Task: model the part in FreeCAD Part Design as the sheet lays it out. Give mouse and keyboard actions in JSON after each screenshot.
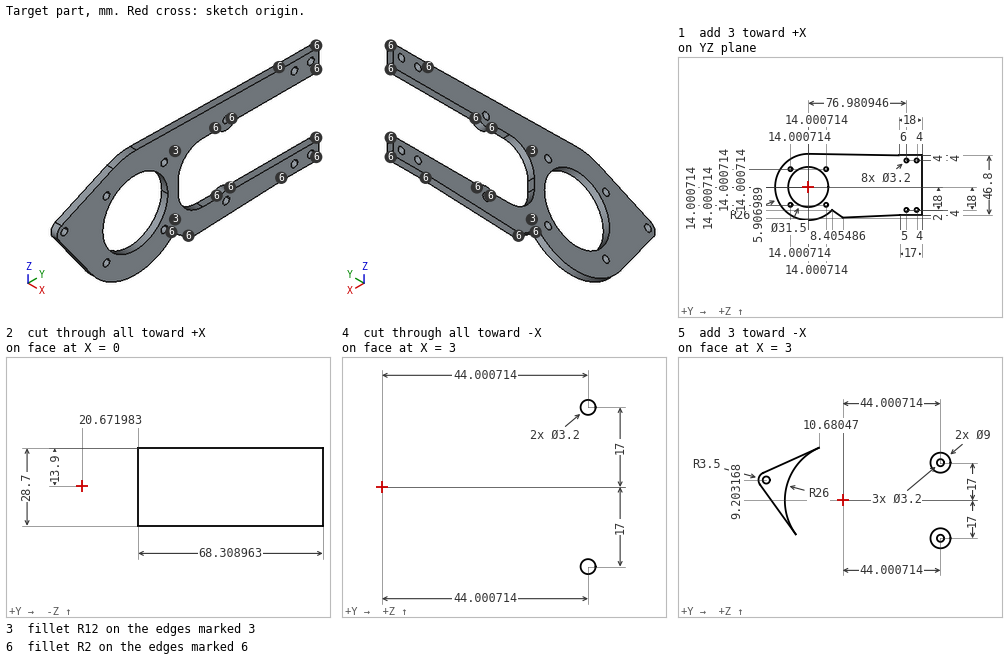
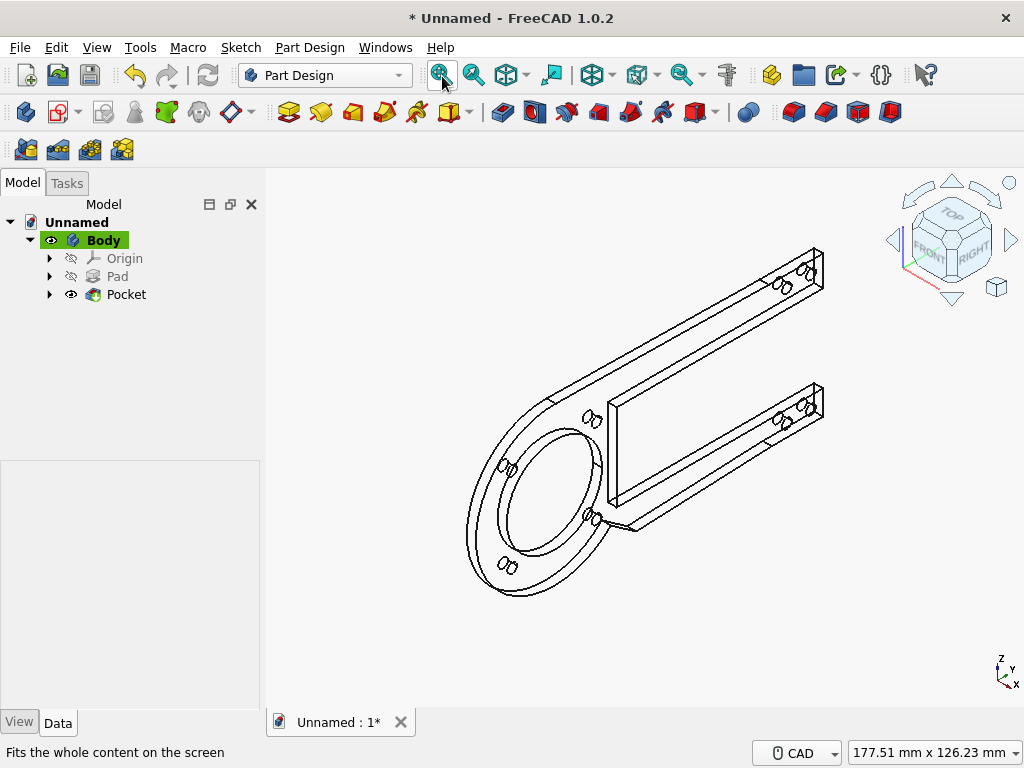
{"action": "left_click", "coordinate": [610, 502]}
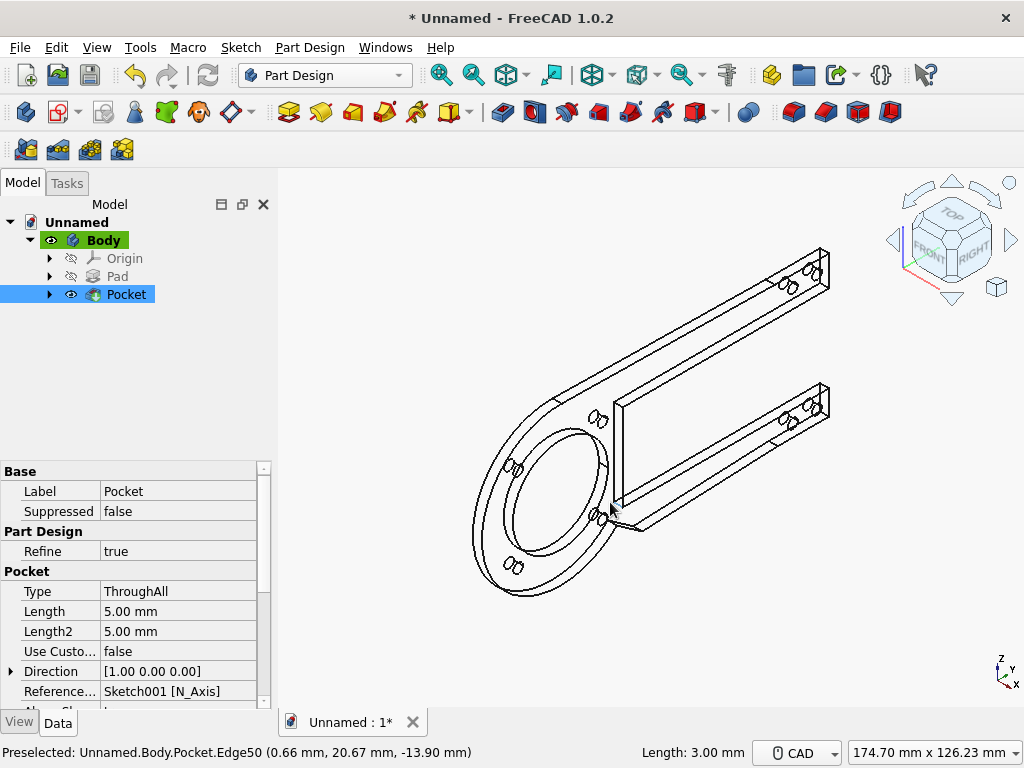
{"action": "left_click", "coordinate": [617, 403], "text": "ctrl"}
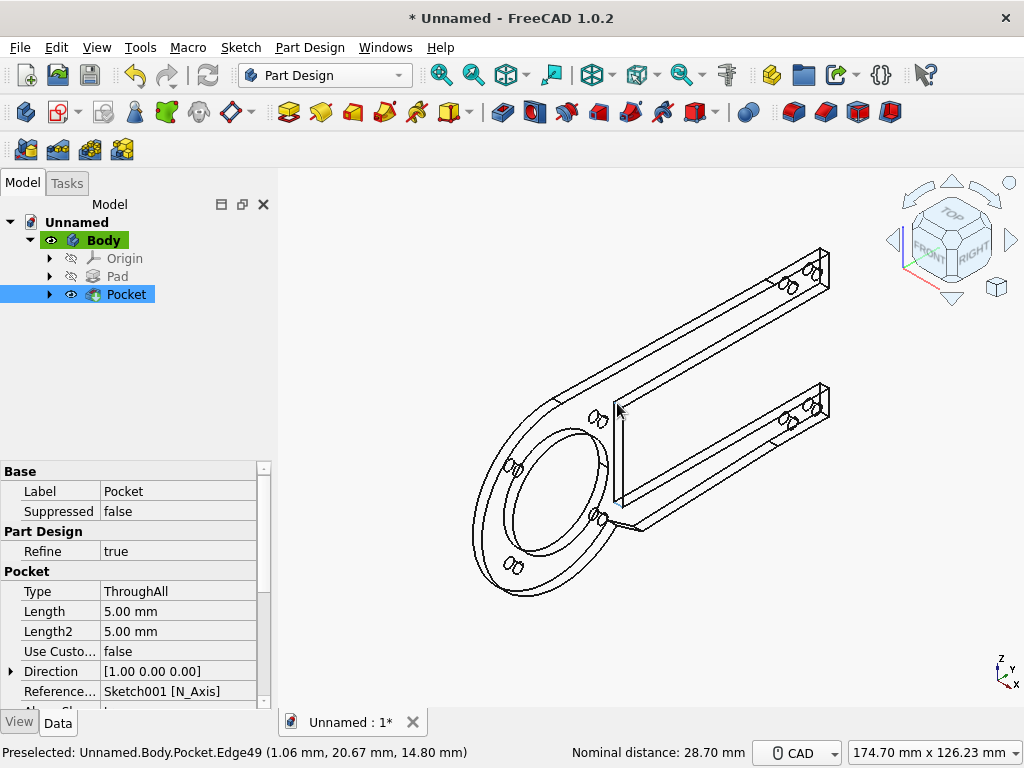
{"action": "key", "text": "v 1"}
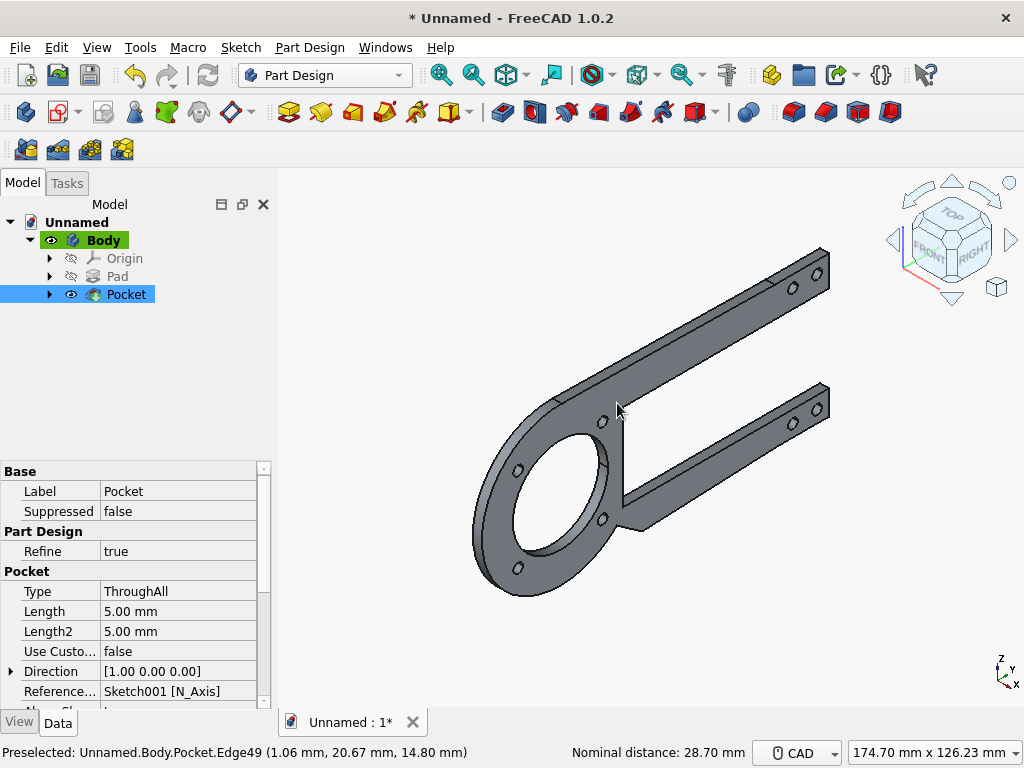
{"action": "left_click", "coordinate": [794, 112]}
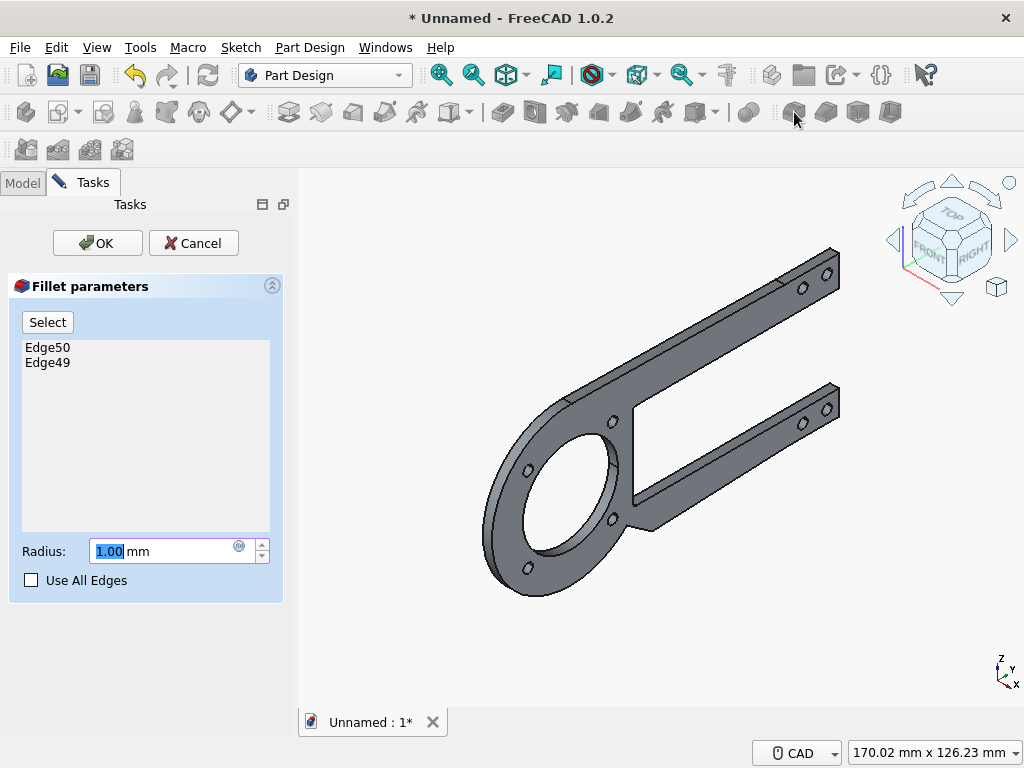
{"action": "type", "text": "12"}
{"action": "key", "text": "Tab"}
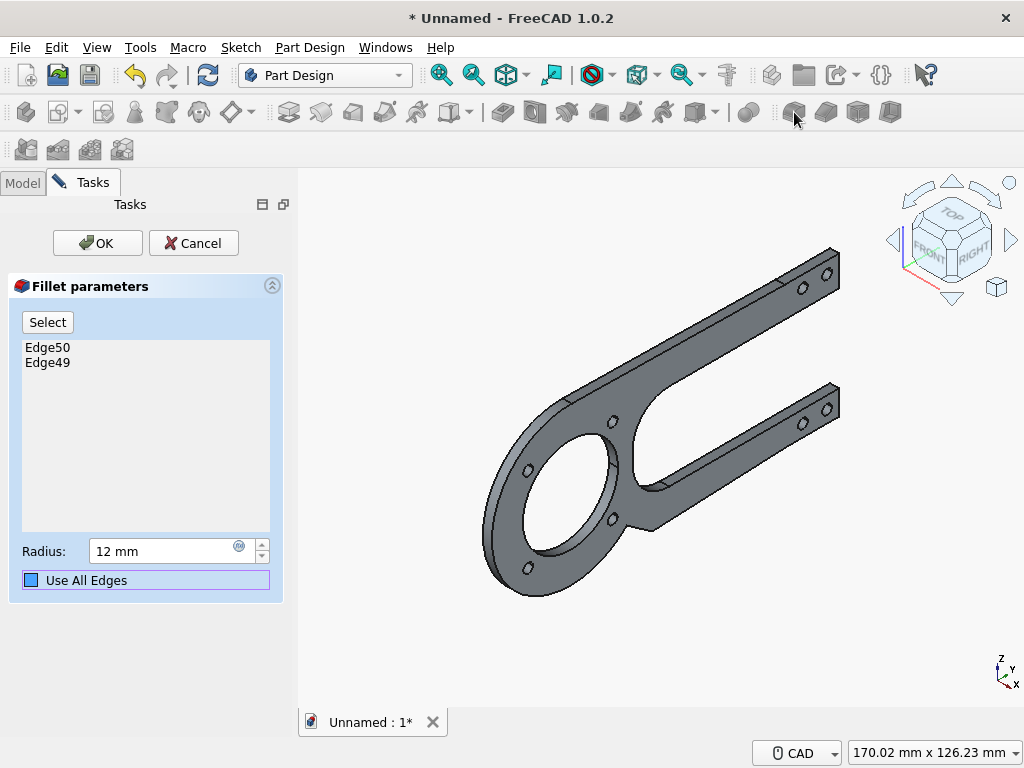
{"action": "left_click", "coordinate": [98, 243]}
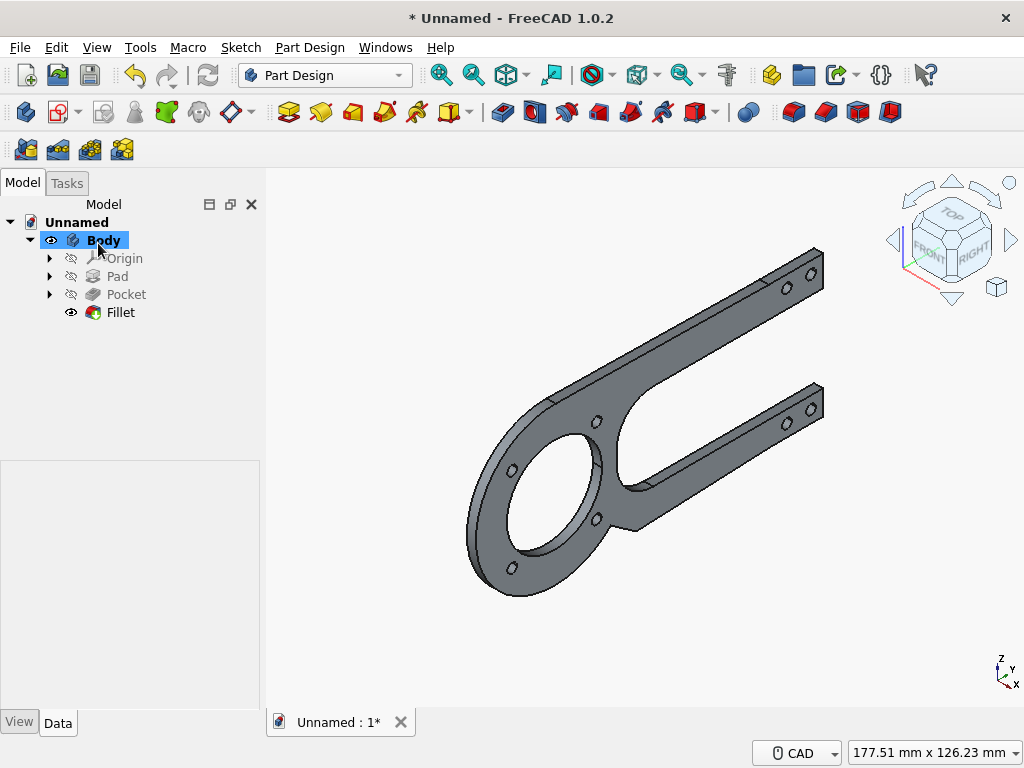
{"action": "left_click", "coordinate": [550, 419]}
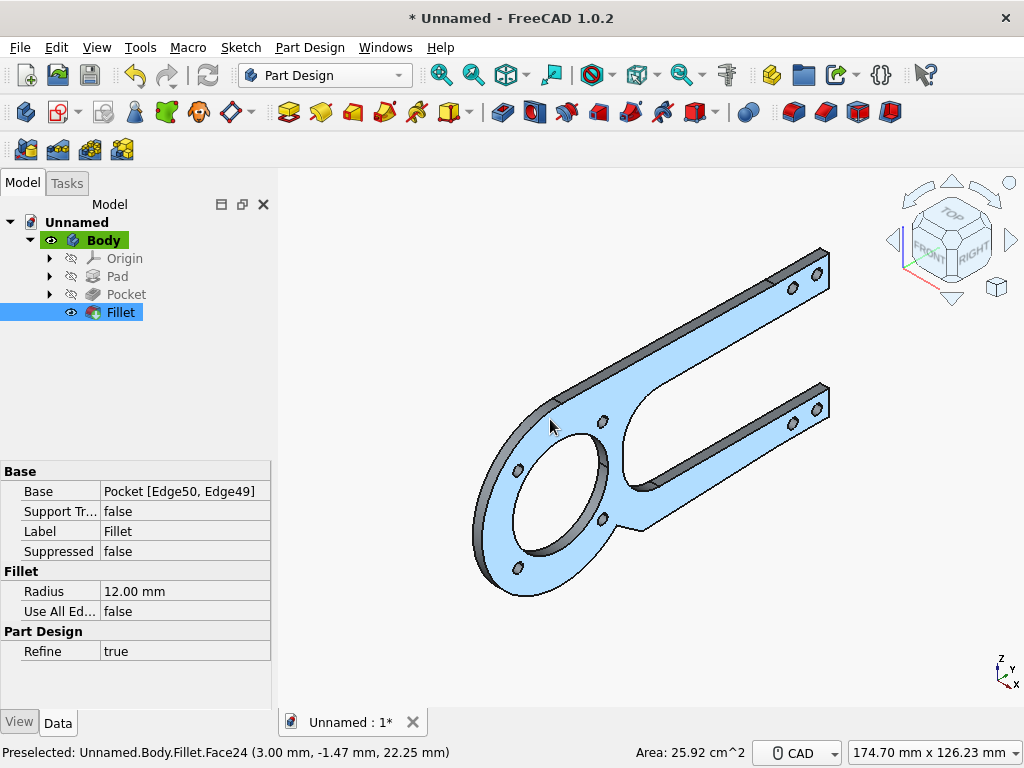
{"action": "left_click", "coordinate": [58, 112]}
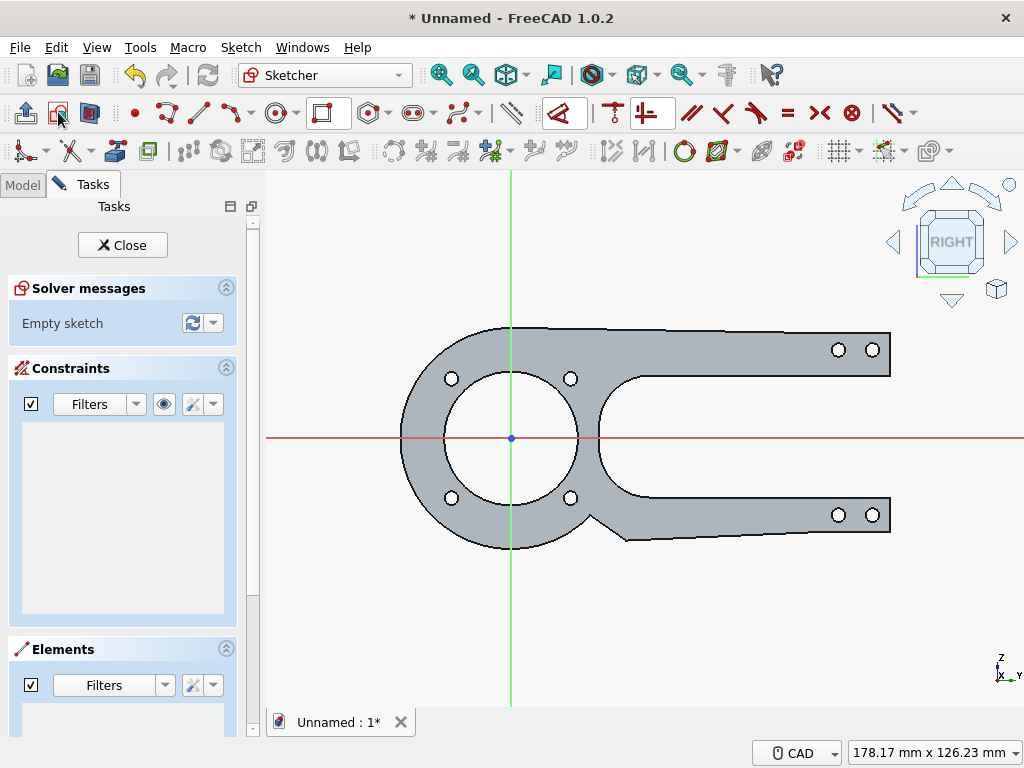
{"action": "scroll", "coordinate": [634, 438], "scroll_direction": "up", "scroll_amount": 4}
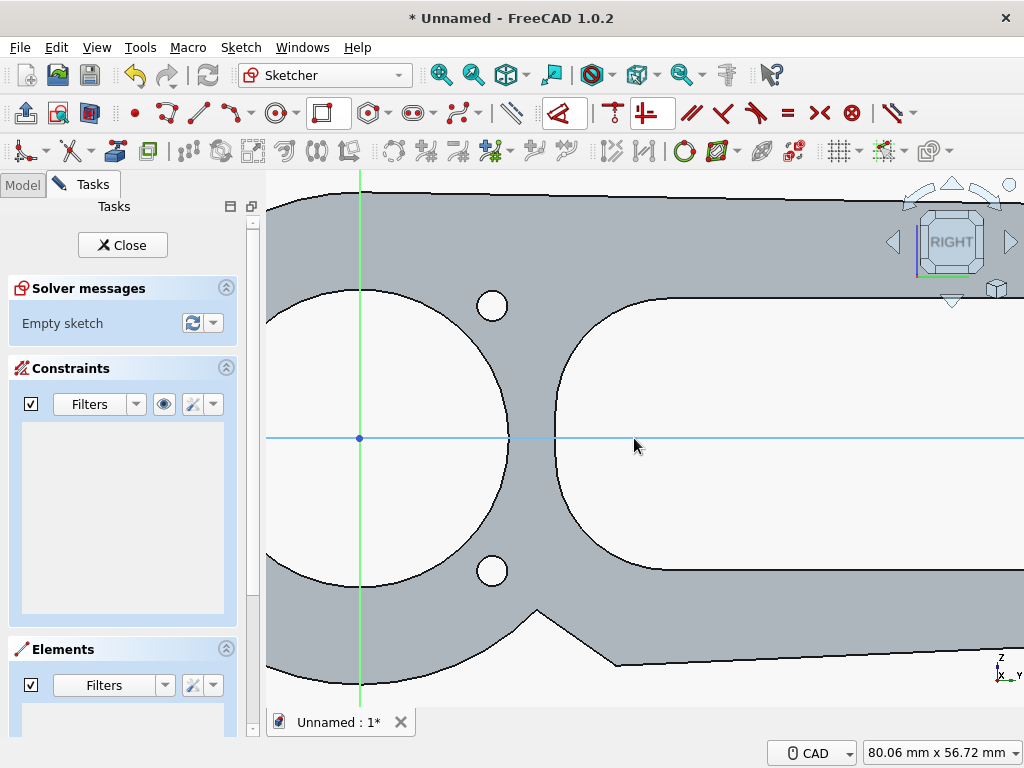
{"action": "left_click", "coordinate": [276, 114]}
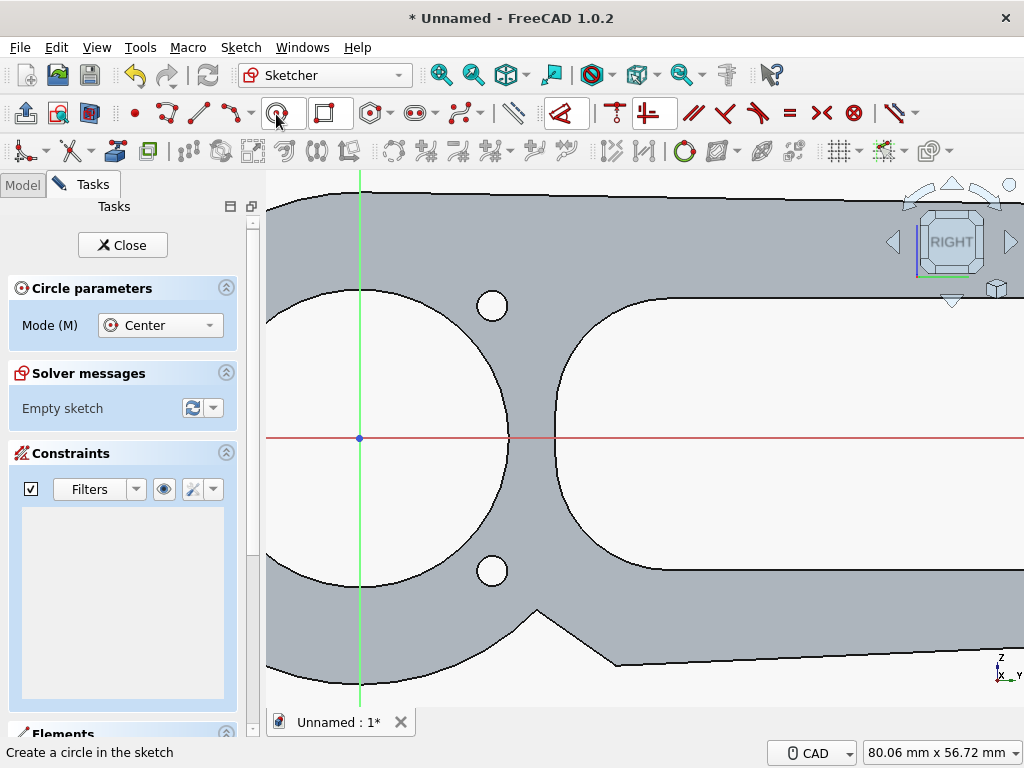
{"action": "scroll", "coordinate": [776, 278], "scroll_direction": "up", "scroll_amount": 3}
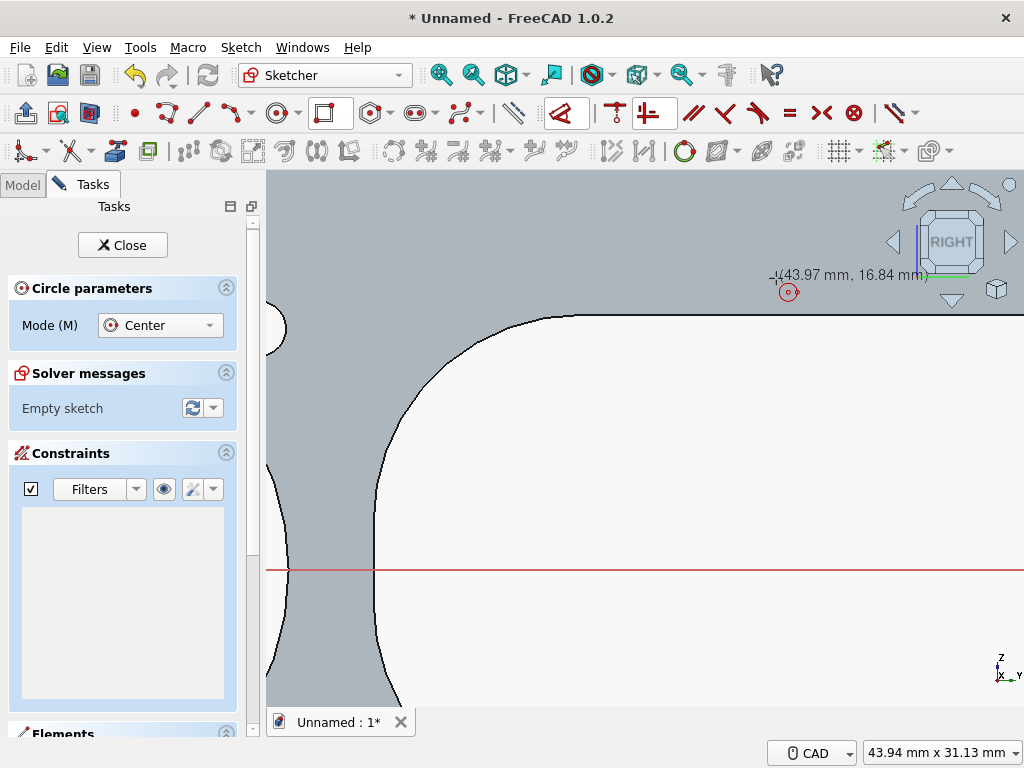
{"action": "left_click", "coordinate": [776, 277]}
{"action": "left_click", "coordinate": [796, 257]}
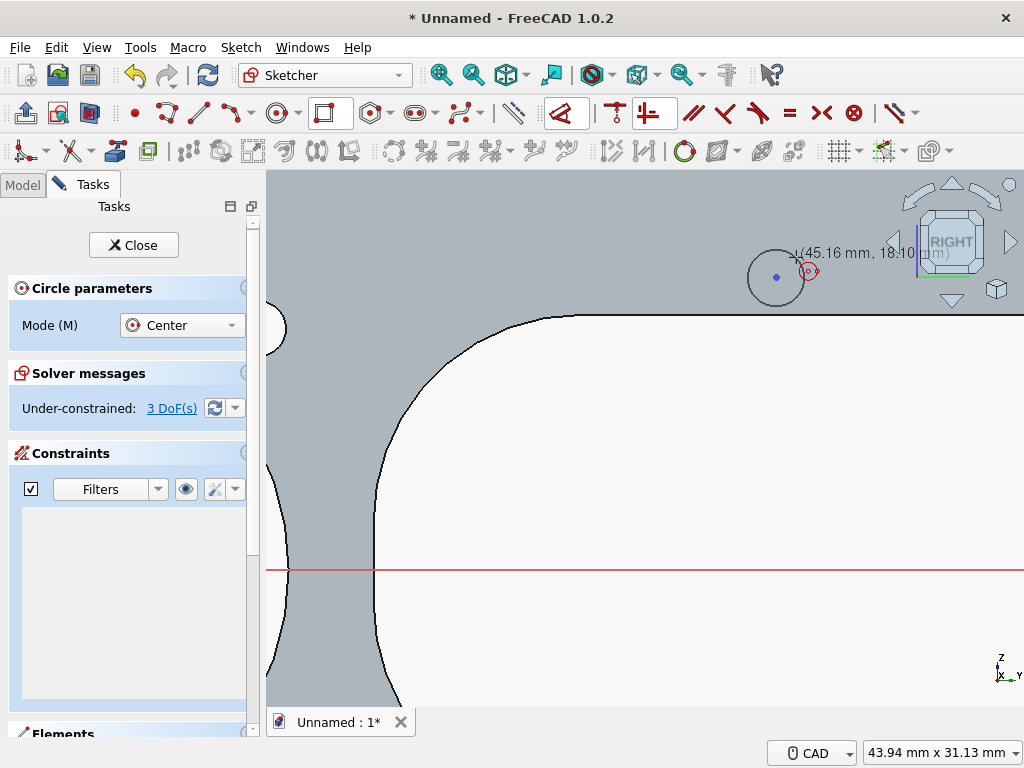
{"action": "scroll", "coordinate": [779, 278], "scroll_direction": "down", "scroll_amount": 3}